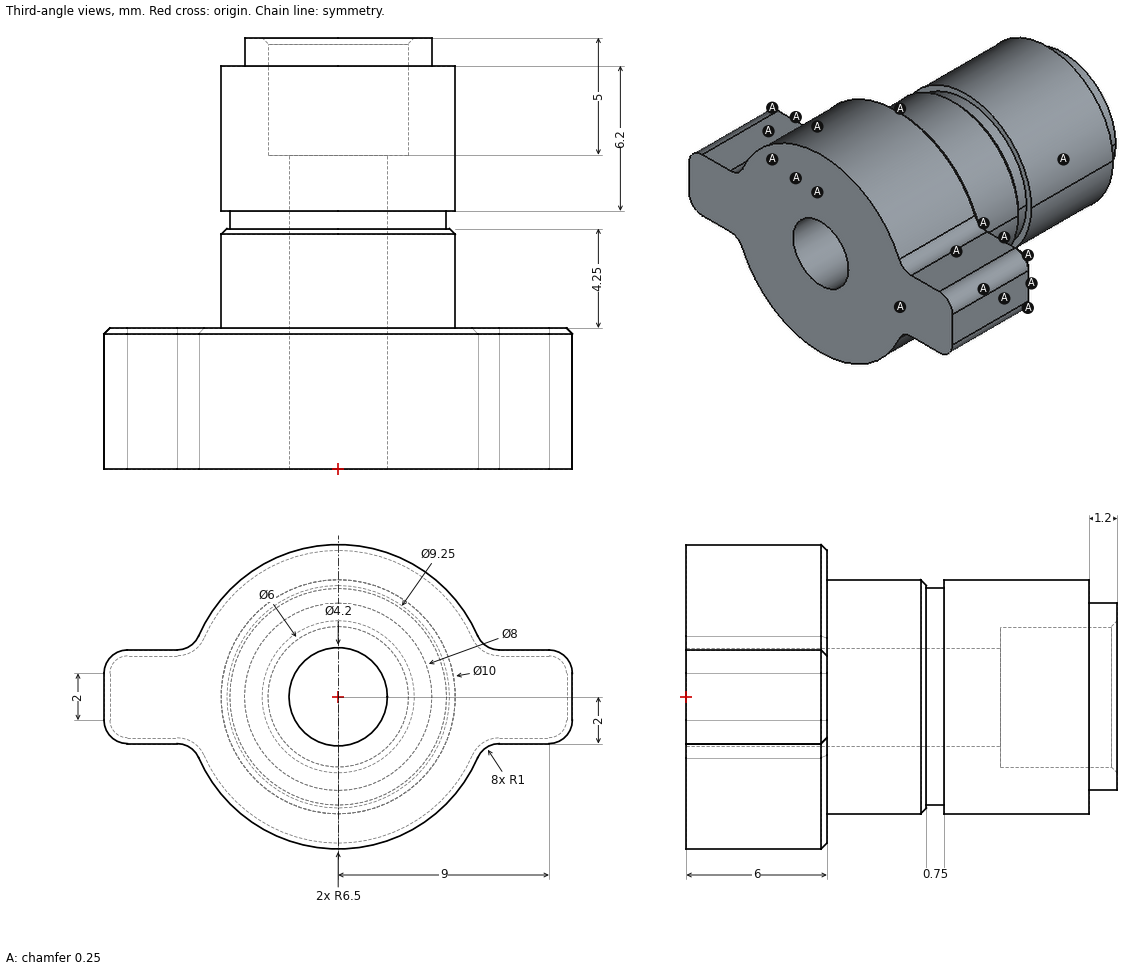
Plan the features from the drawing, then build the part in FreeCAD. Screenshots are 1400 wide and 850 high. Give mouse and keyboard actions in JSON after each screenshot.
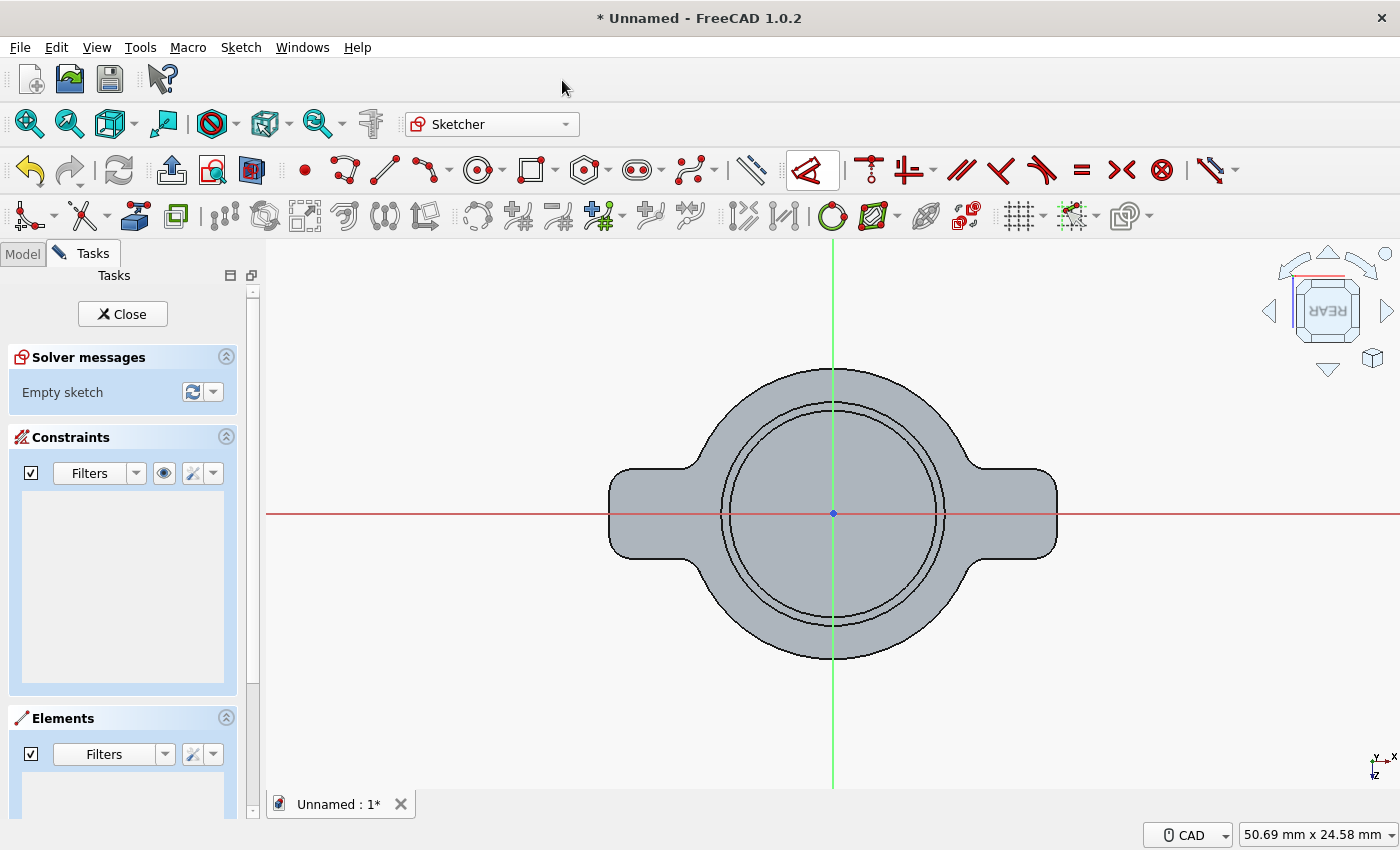
{"action": "scroll", "coordinate": [972, 514], "scroll_direction": "up", "scroll_amount": 2}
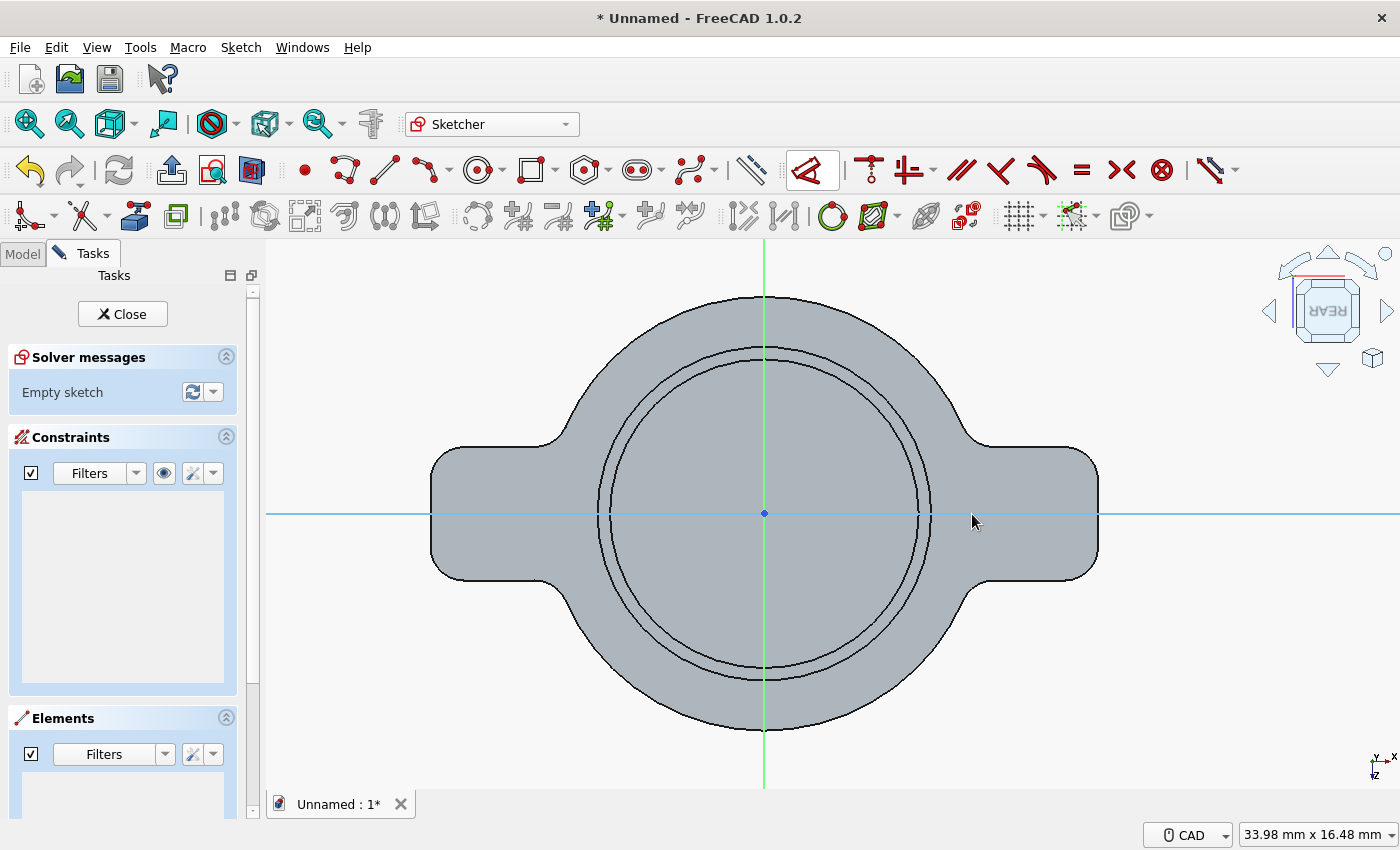
{"action": "left_click", "coordinate": [478, 170]}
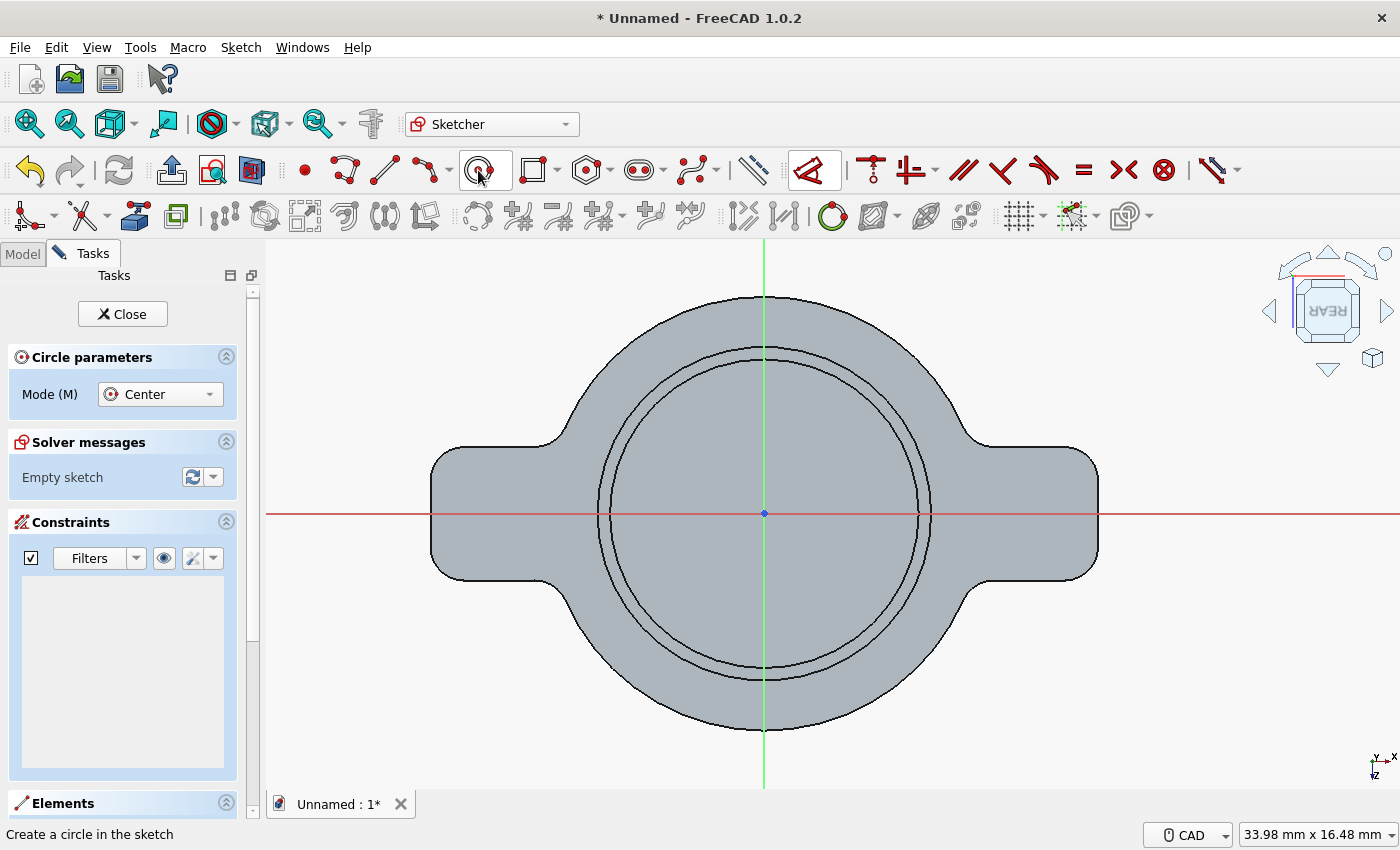
{"action": "left_click", "coordinate": [764, 514]}
{"action": "mouse_move", "coordinate": [882, 396]}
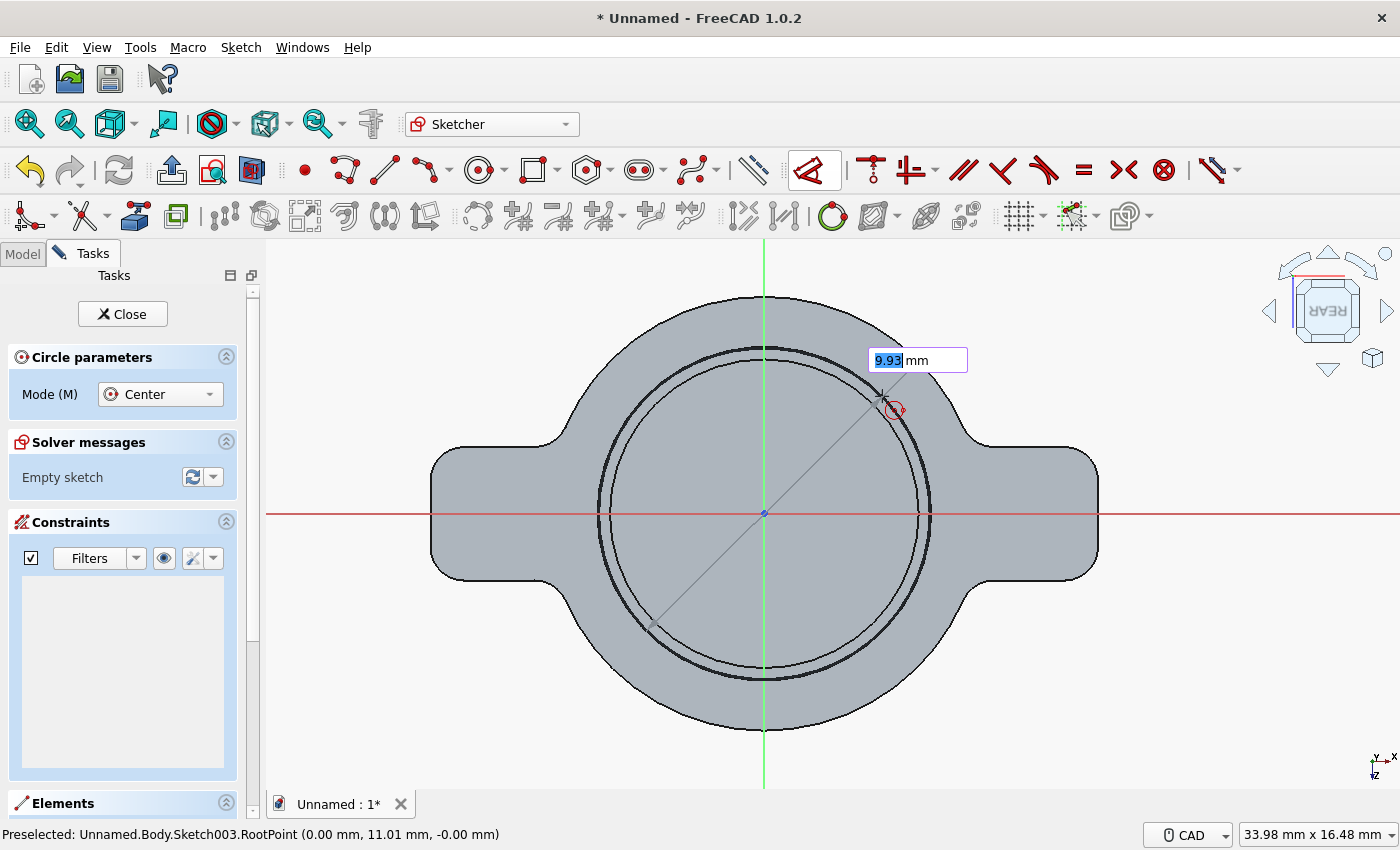
{"action": "type", "text": "10"}
{"action": "key", "text": "Return"}
{"action": "key", "text": "Escape"}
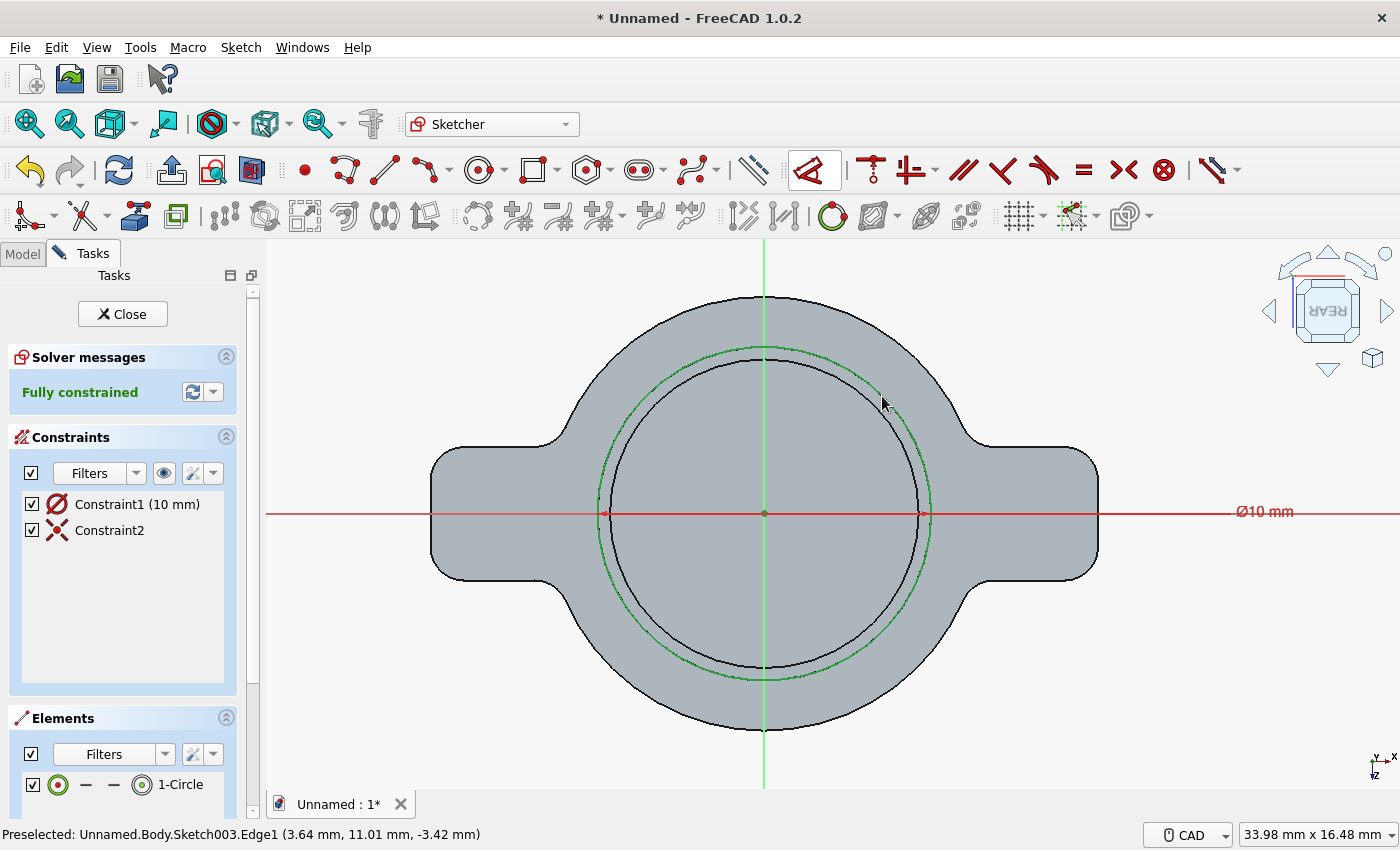
{"action": "left_click", "coordinate": [123, 314]}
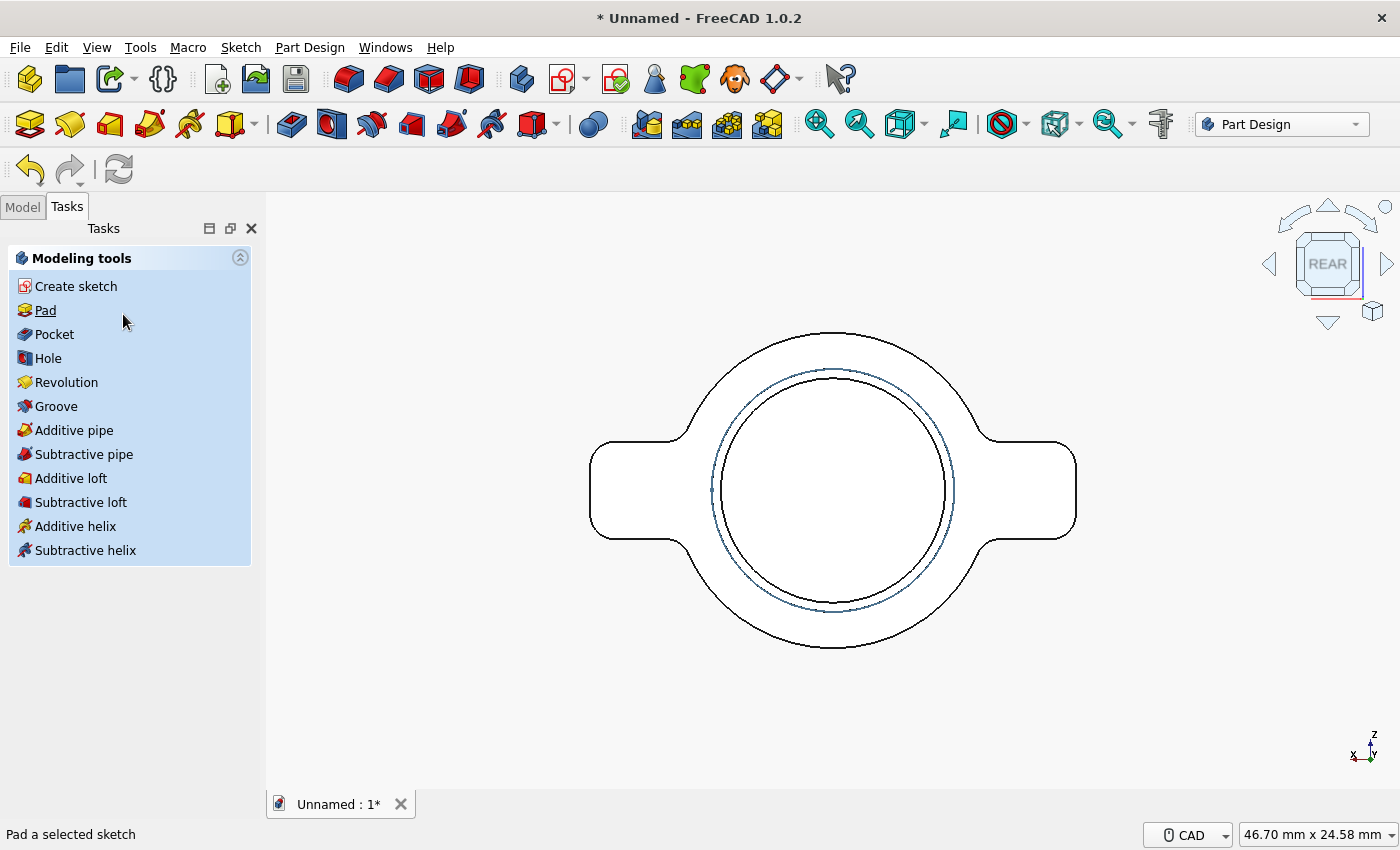
{"action": "left_click", "coordinate": [30, 124]}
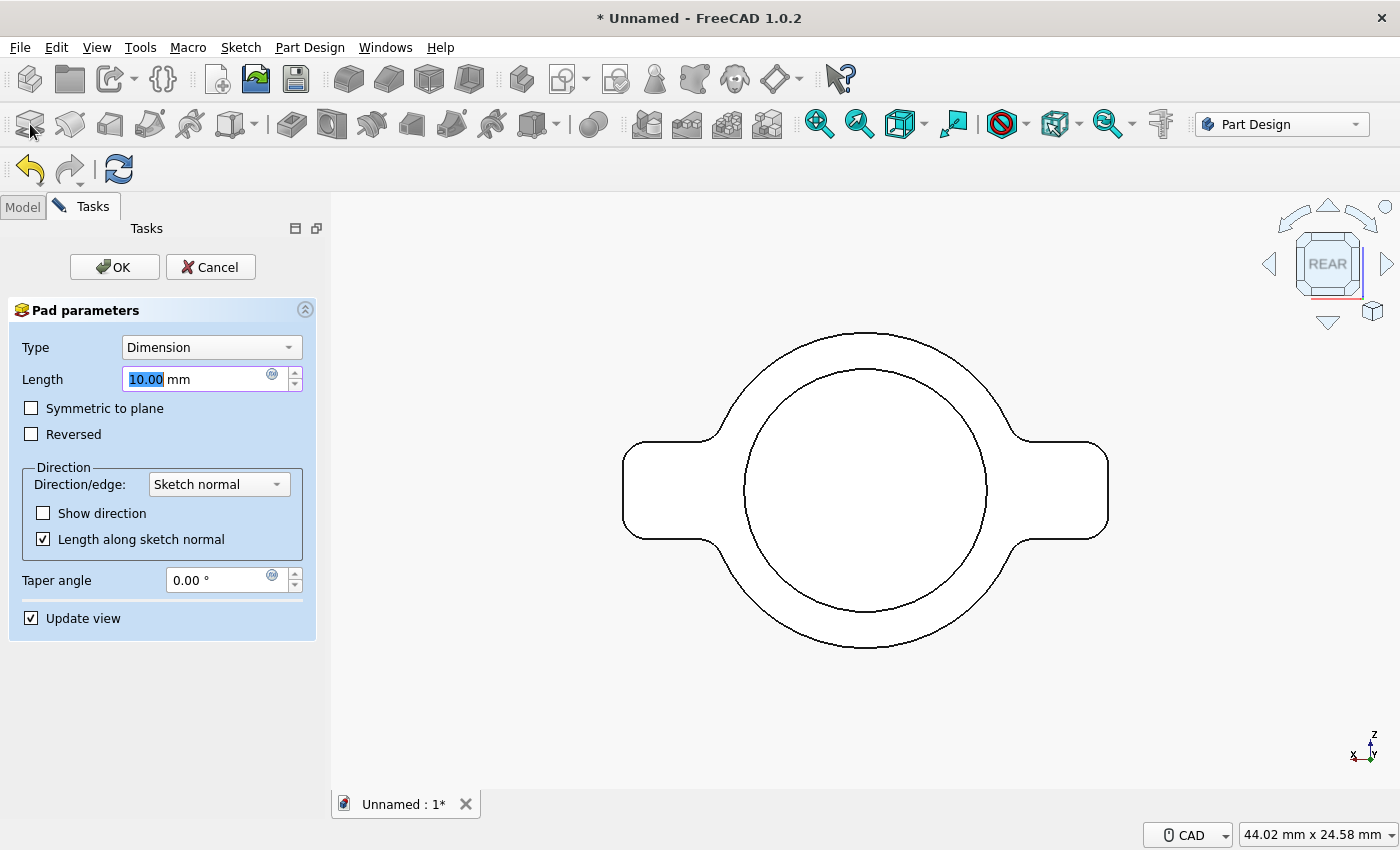
{"action": "type", "text": "6.2"}
{"action": "key", "text": "Tab"}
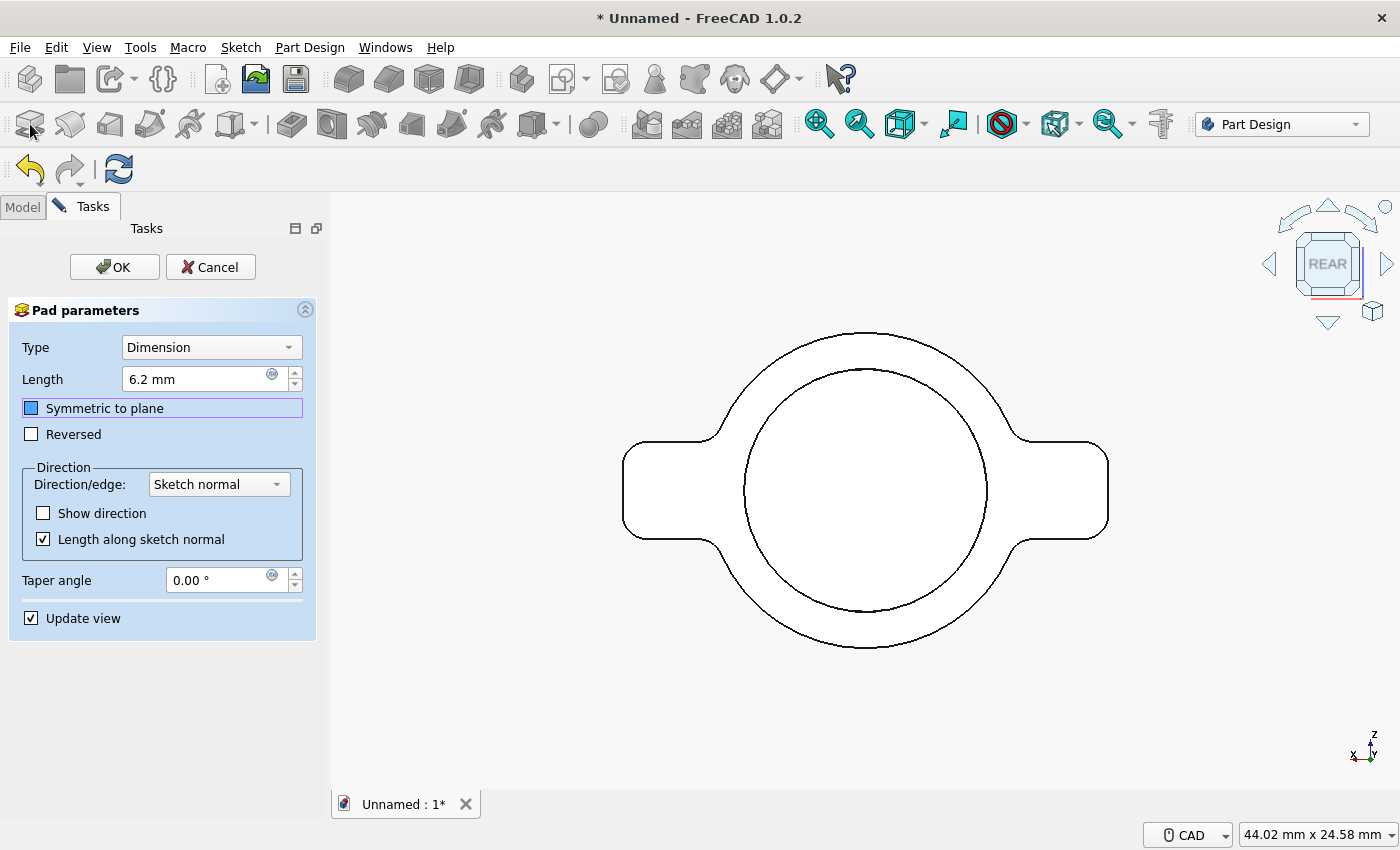
{"action": "left_click", "coordinate": [115, 267]}